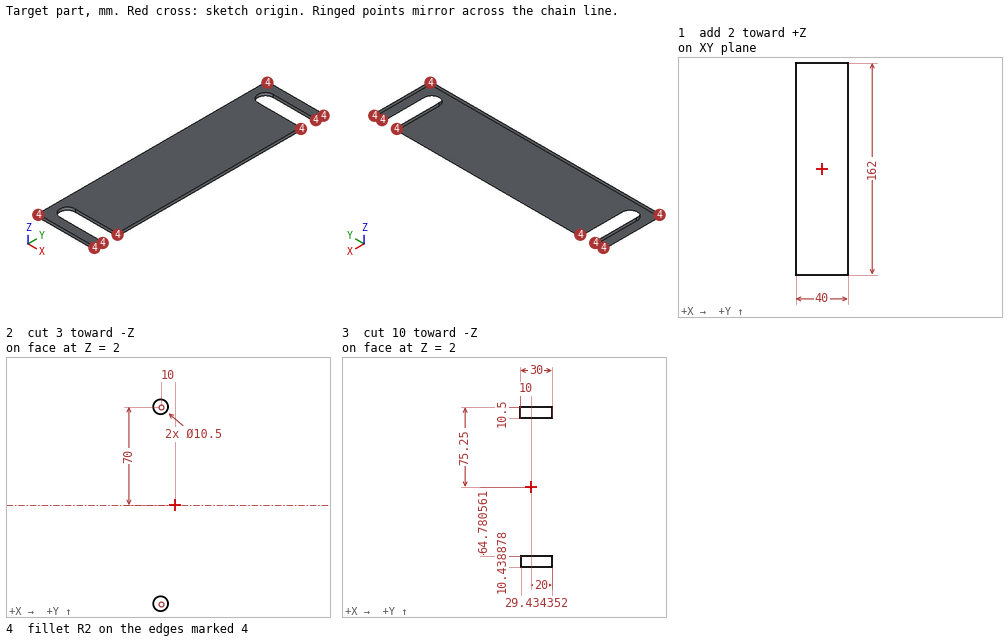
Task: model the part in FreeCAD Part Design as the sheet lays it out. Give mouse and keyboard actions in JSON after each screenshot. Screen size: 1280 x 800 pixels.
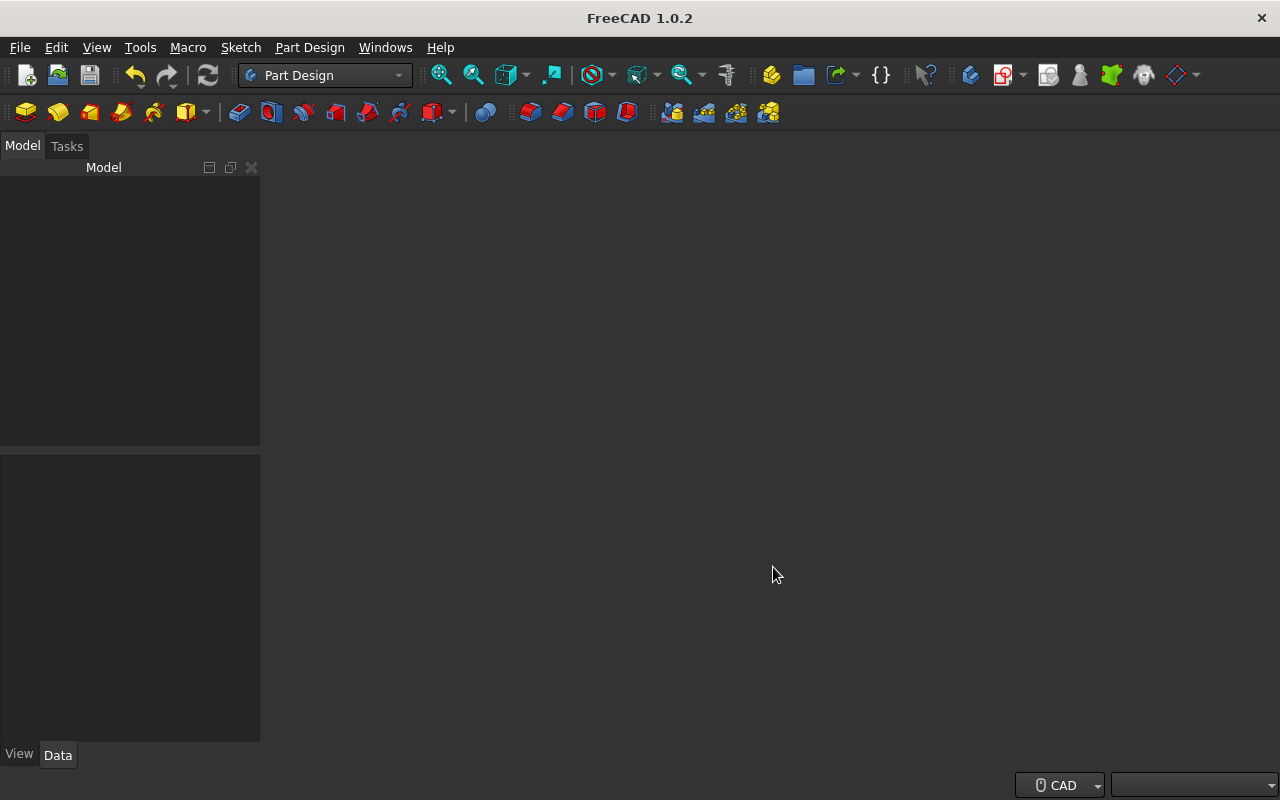
{"action": "left_click", "coordinate": [26, 76]}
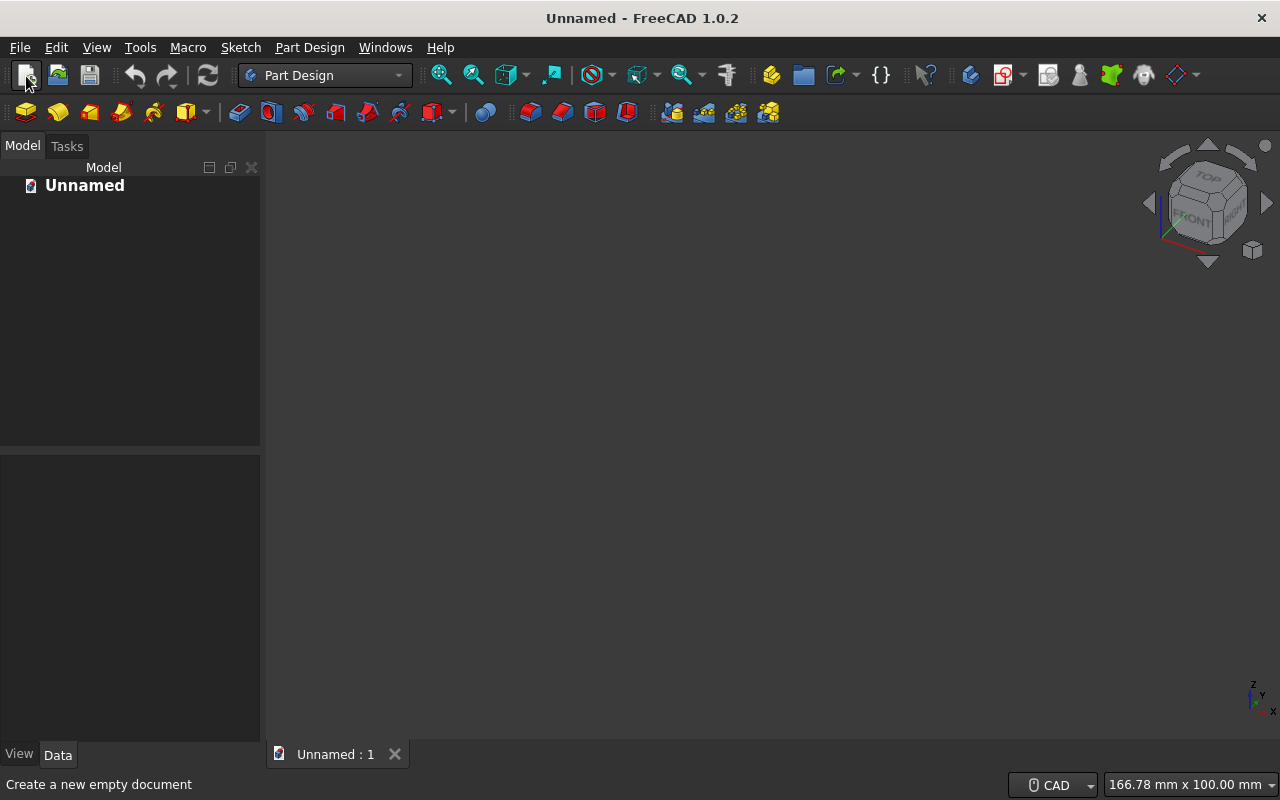
{"action": "left_click", "coordinate": [1004, 76]}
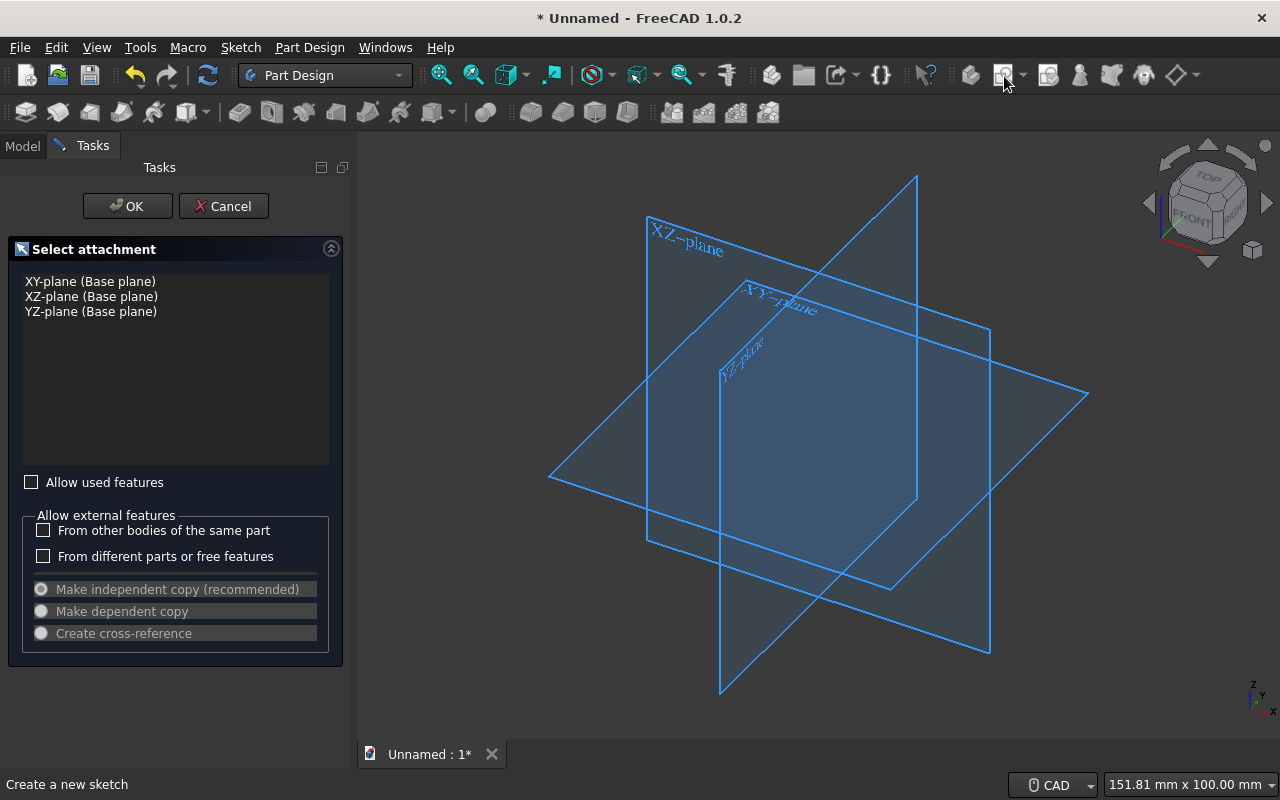
{"action": "left_click", "coordinate": [82, 282]}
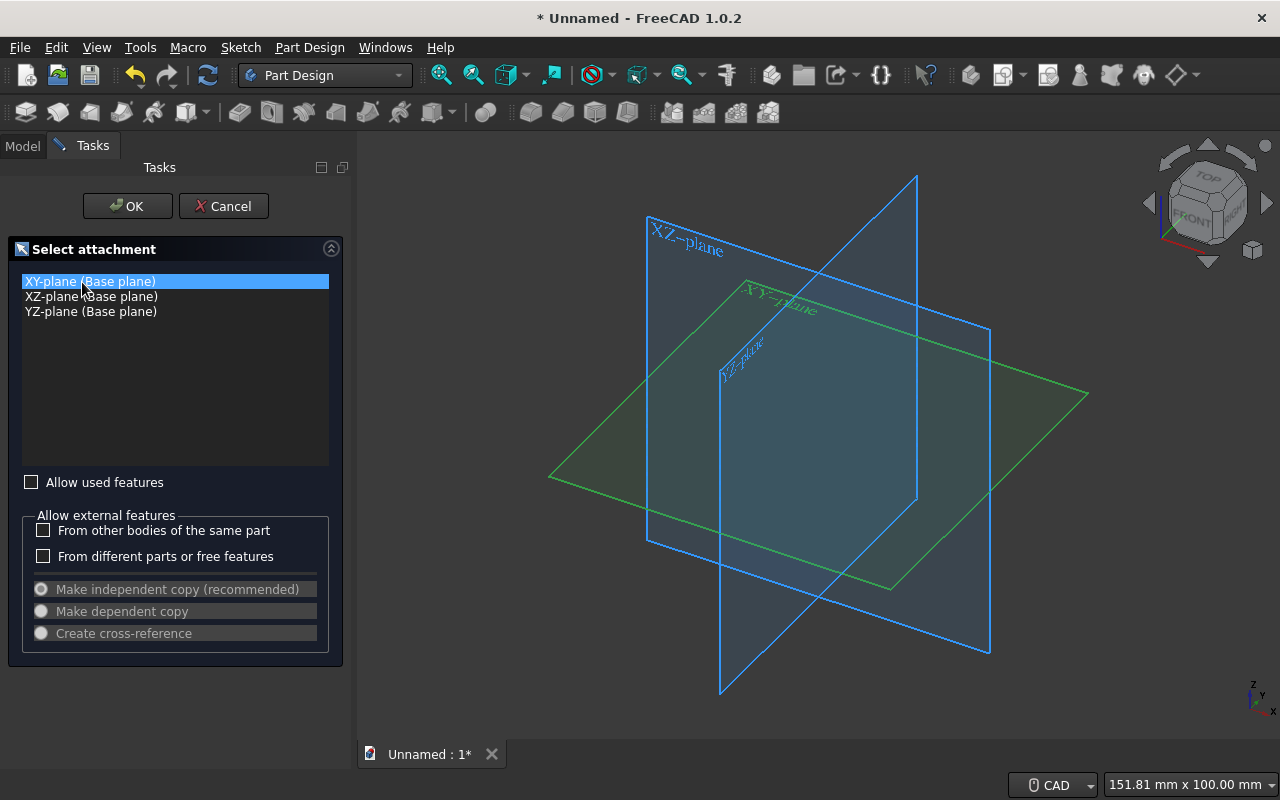
{"action": "left_click", "coordinate": [128, 206]}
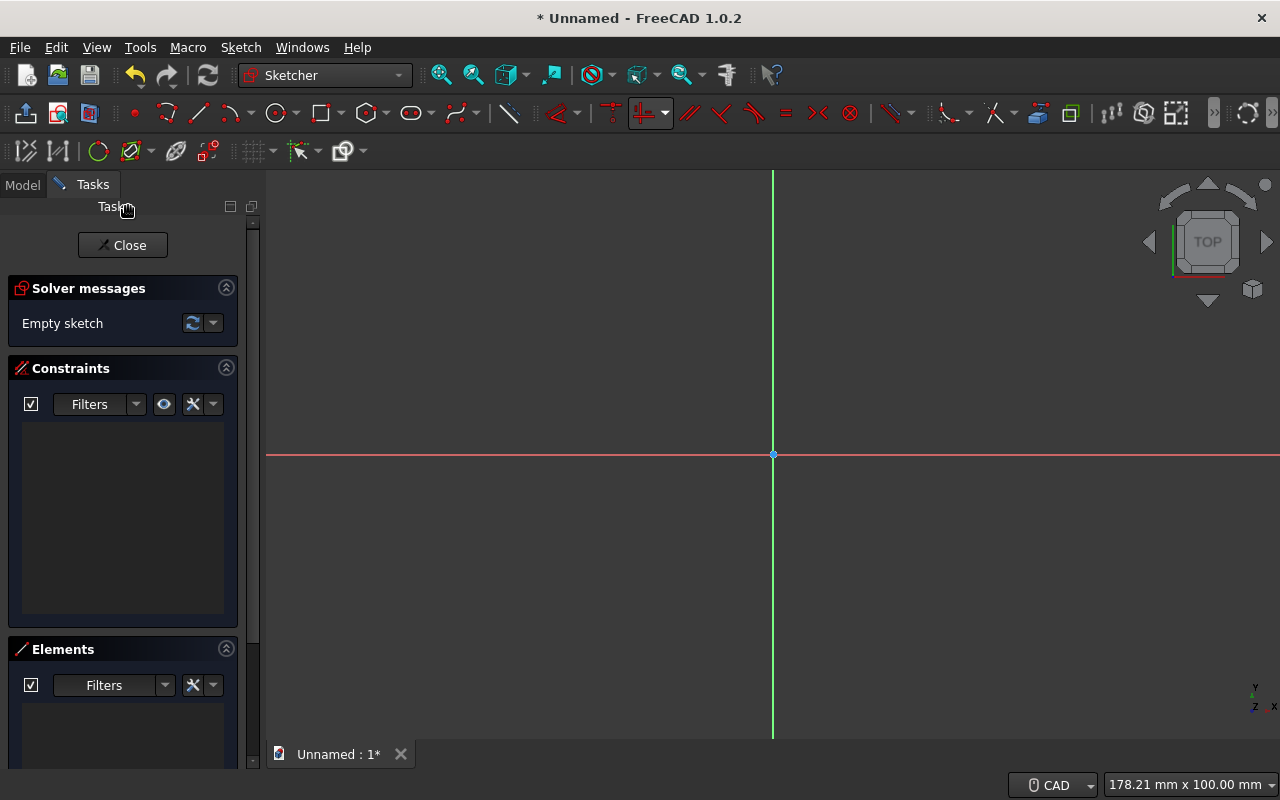
{"action": "scroll", "coordinate": [665, 454], "scroll_direction": "down", "scroll_amount": 5}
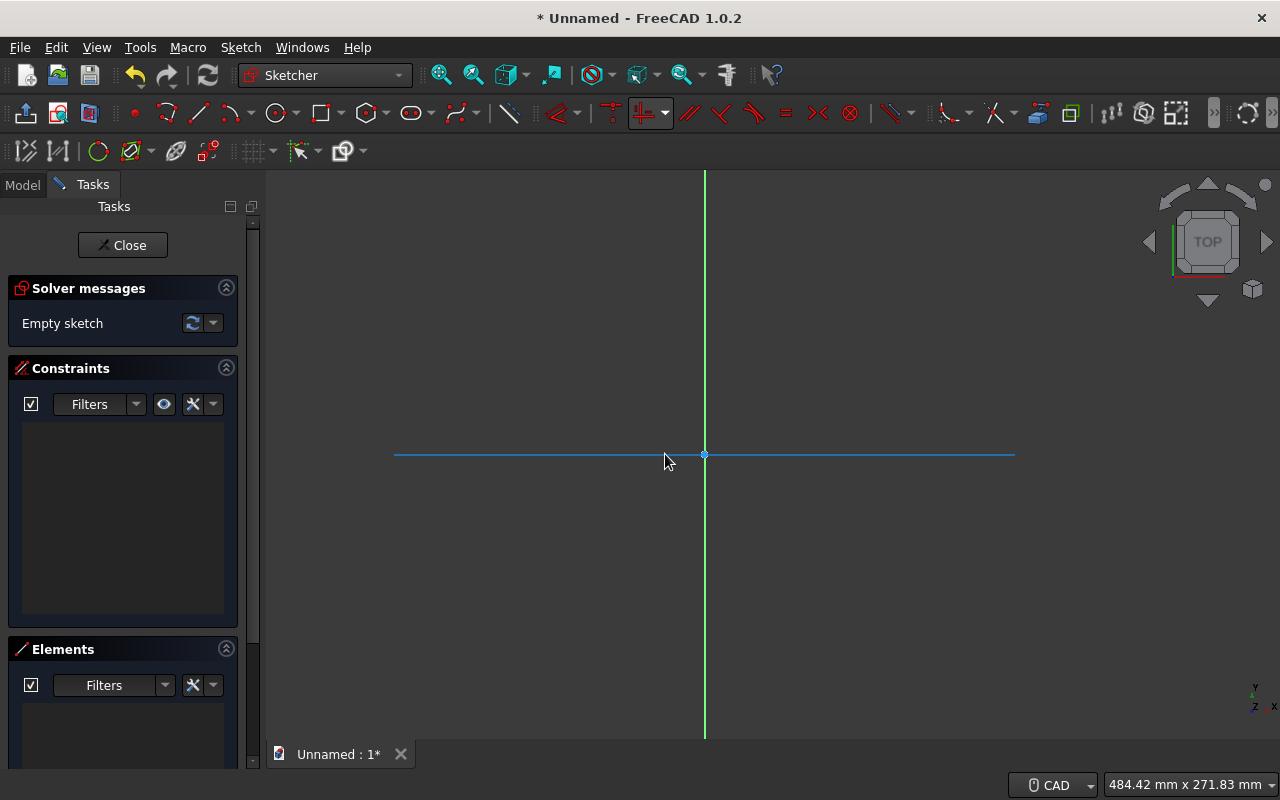
{"action": "left_click", "coordinate": [344, 114]}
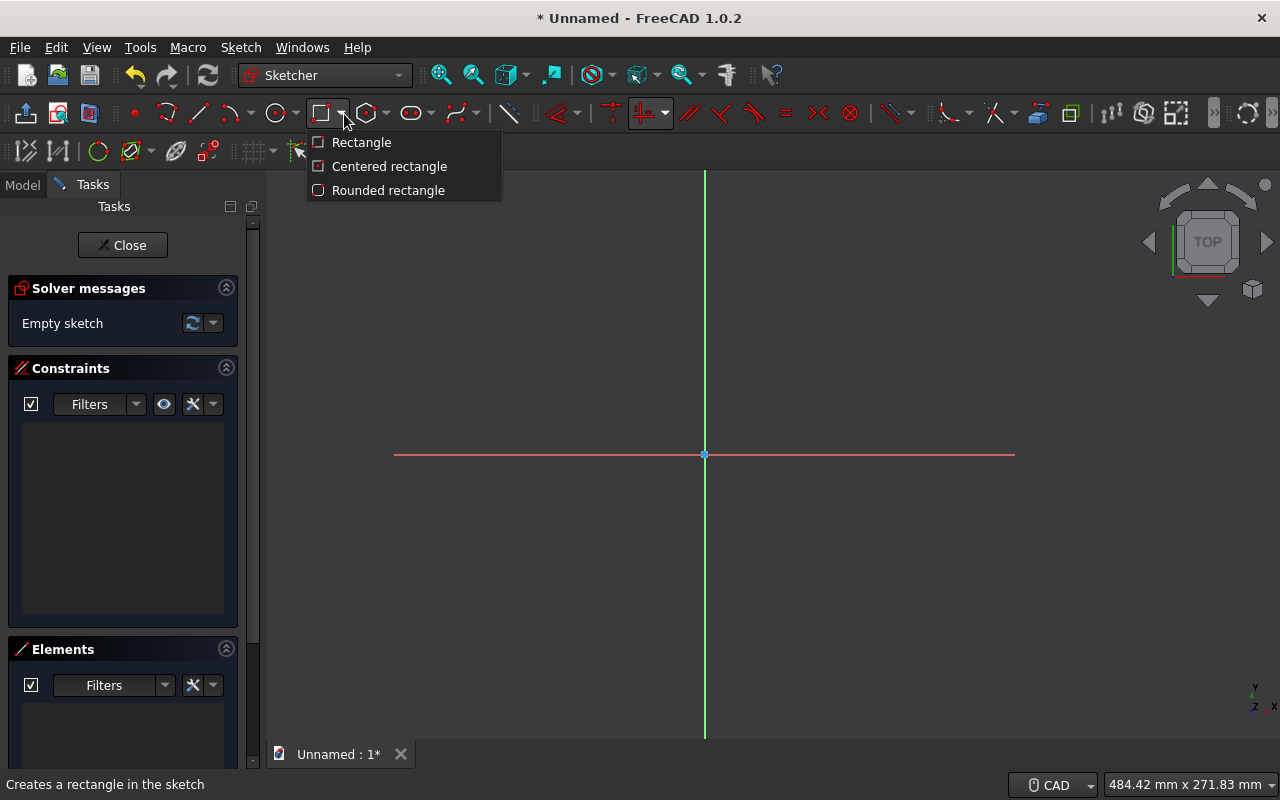
{"action": "left_click", "coordinate": [404, 166]}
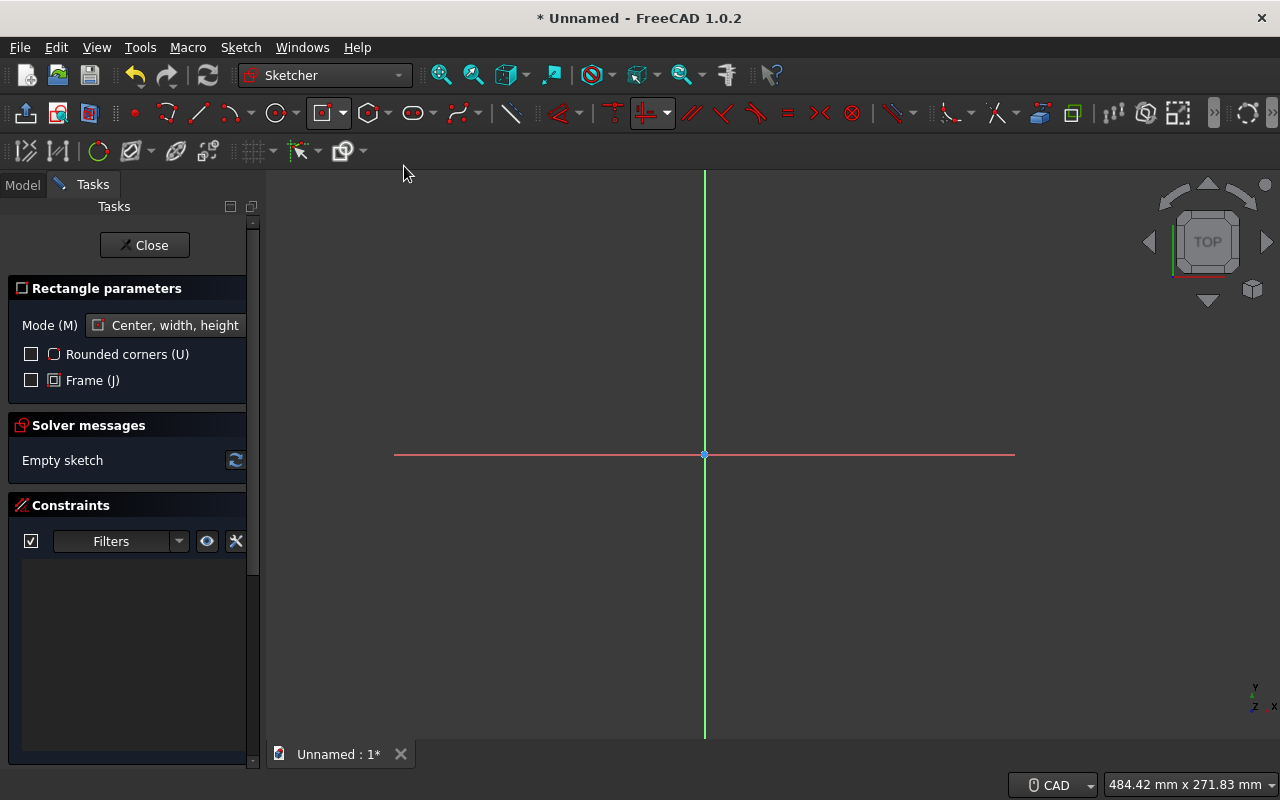
{"action": "left_click", "coordinate": [705, 454]}
{"action": "left_click", "coordinate": [747, 285]}
{"action": "key", "text": "Escape"}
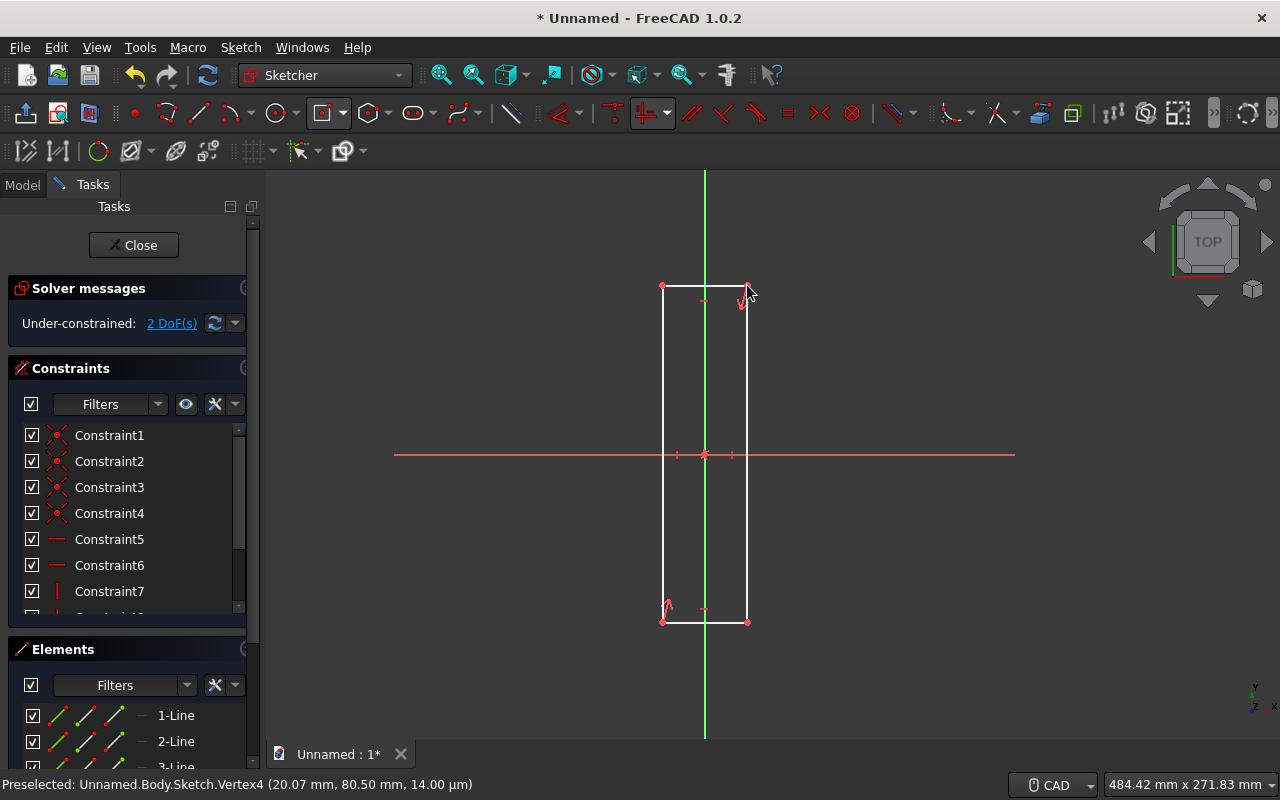
{"action": "left_click", "coordinate": [558, 114]}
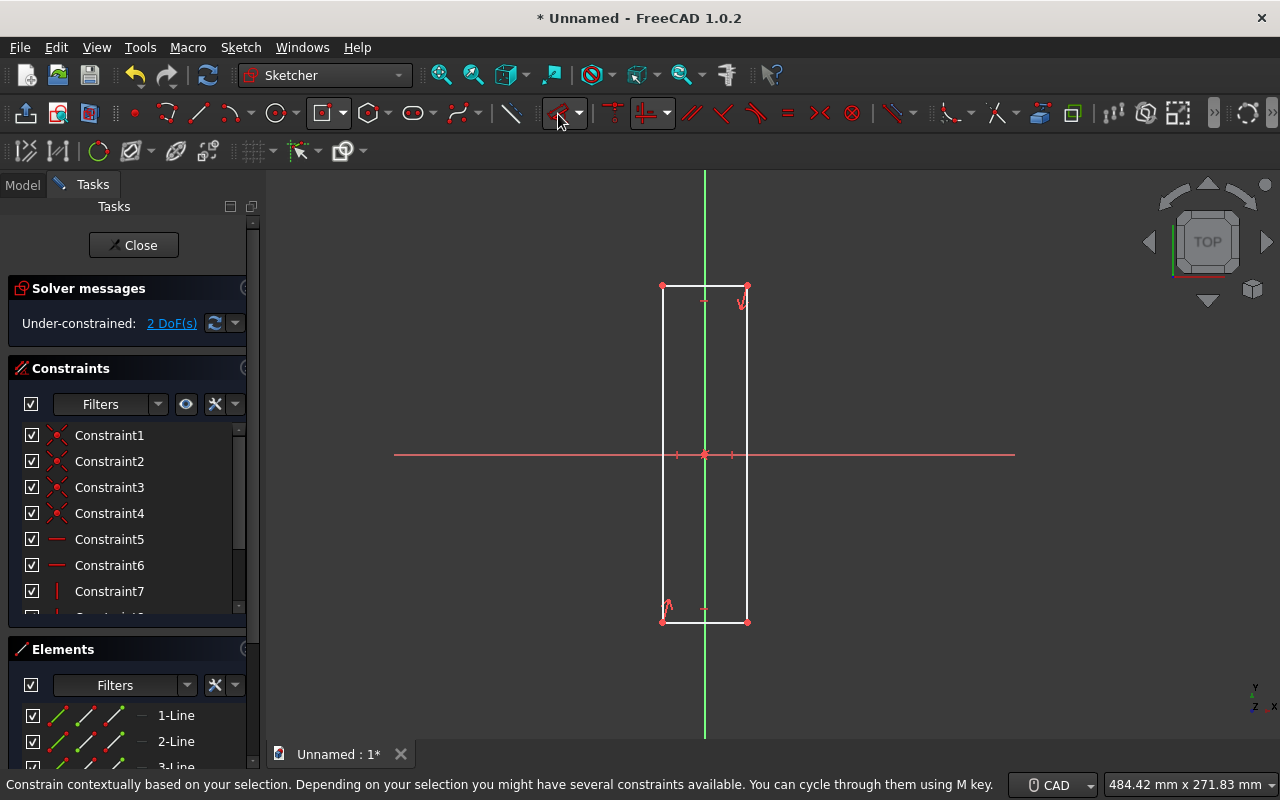
{"action": "left_click", "coordinate": [688, 623]}
{"action": "left_click", "coordinate": [686, 657]}